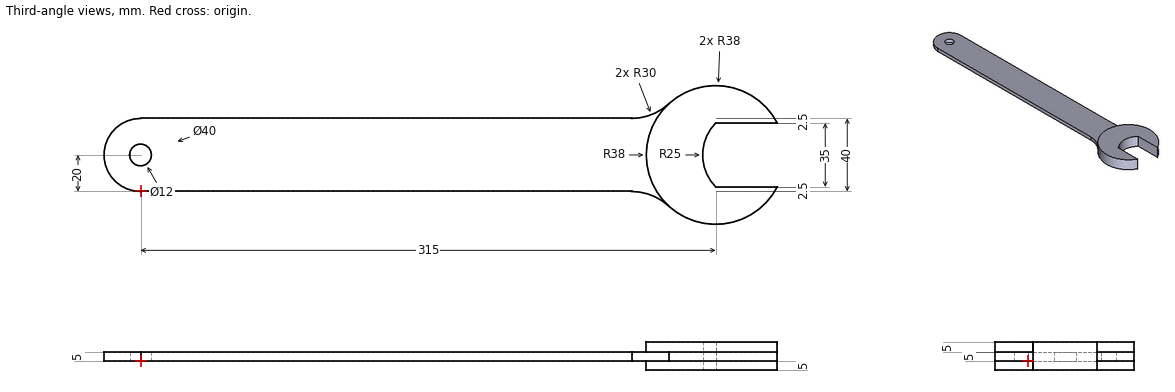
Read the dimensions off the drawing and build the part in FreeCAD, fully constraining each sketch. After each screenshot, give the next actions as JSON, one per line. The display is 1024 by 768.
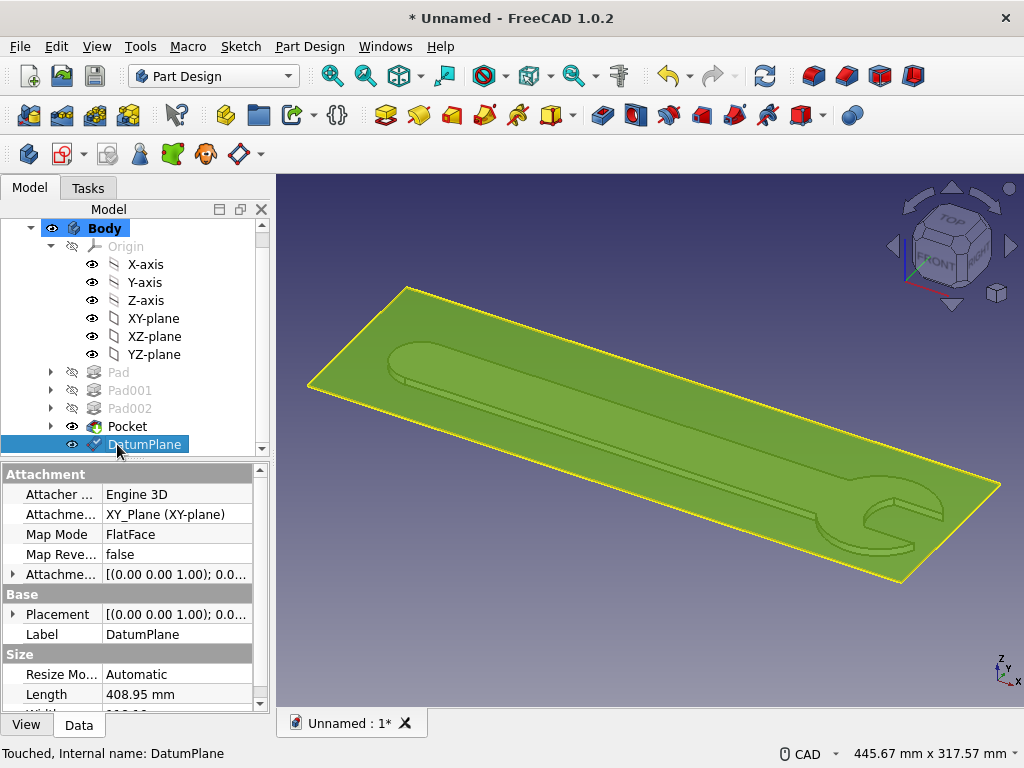
{"action": "left_click", "coordinate": [62, 154]}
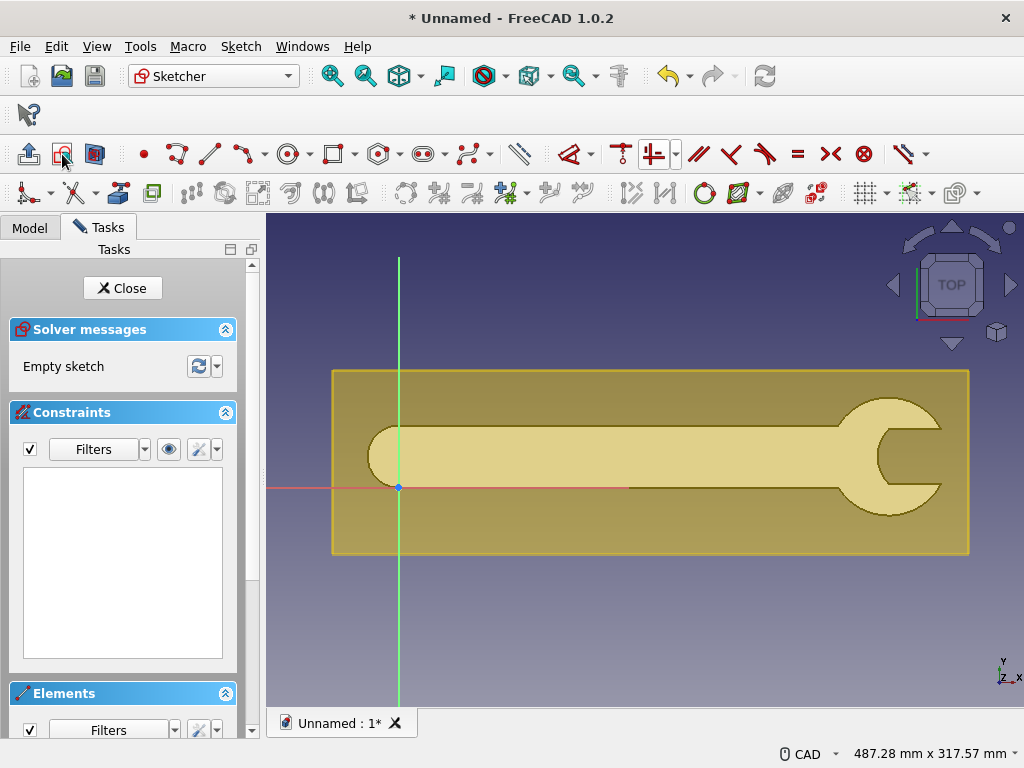
{"action": "scroll", "coordinate": [576, 460], "scroll_direction": "down", "scroll_amount": 5}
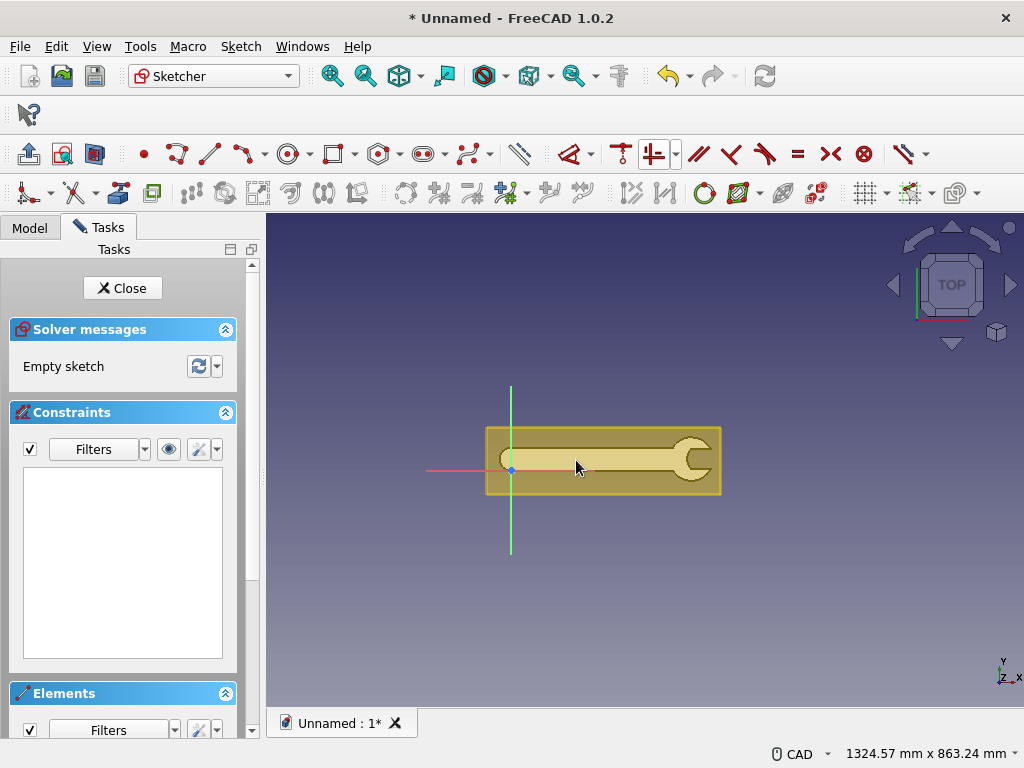
{"action": "scroll", "coordinate": [704, 459], "scroll_direction": "up", "scroll_amount": 11}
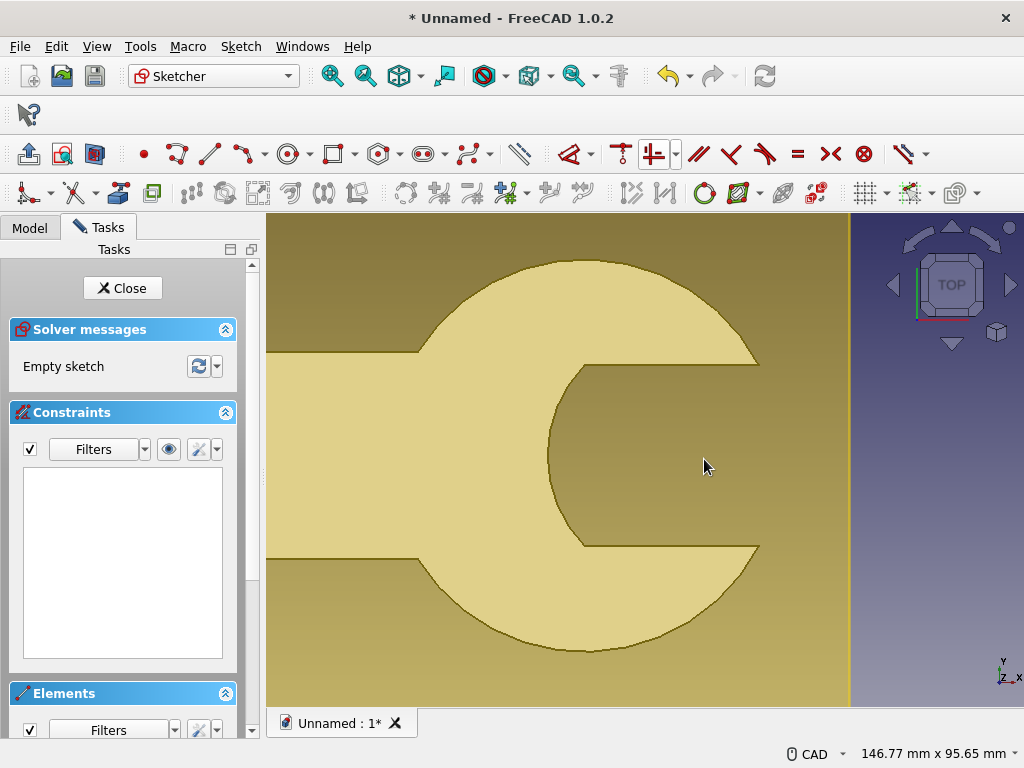
{"action": "left_click", "coordinate": [210, 154]}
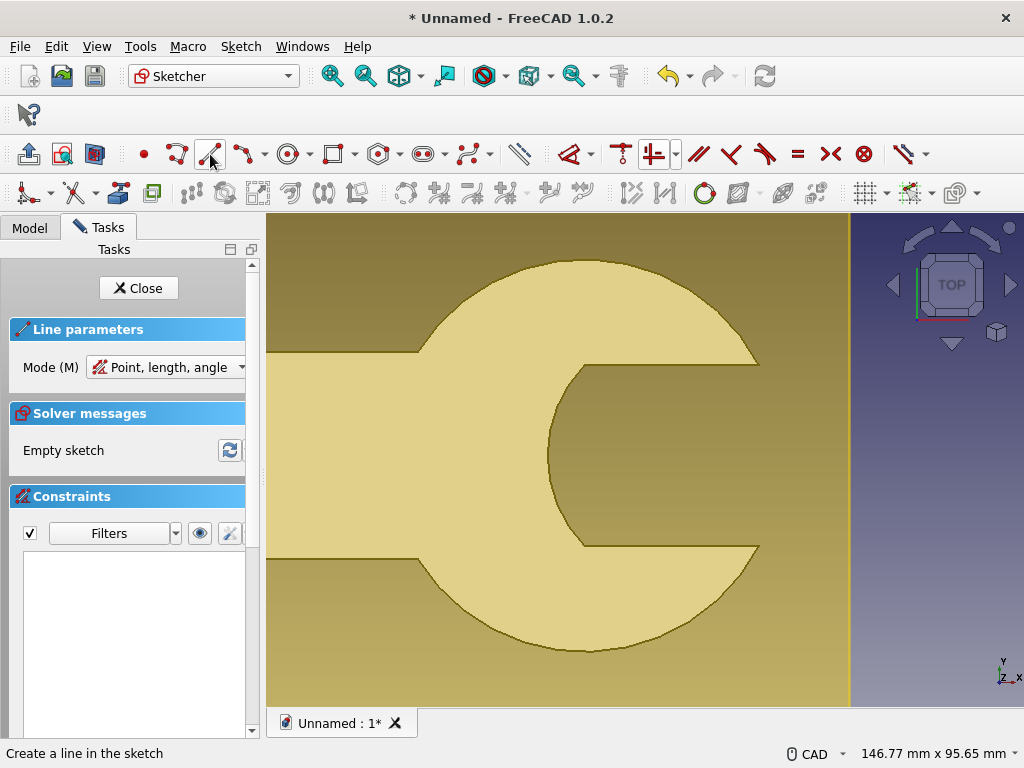
{"action": "left_click", "coordinate": [585, 365]}
{"action": "left_click", "coordinate": [759, 365]}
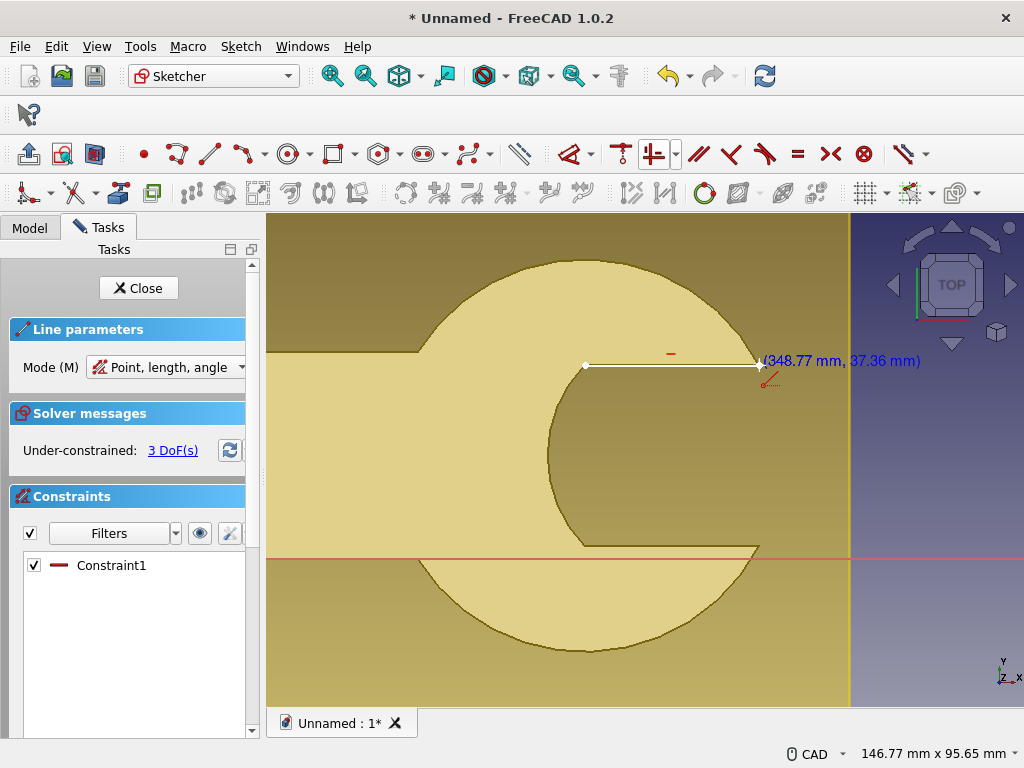
{"action": "scroll", "coordinate": [759, 546], "scroll_direction": "up", "scroll_amount": 2}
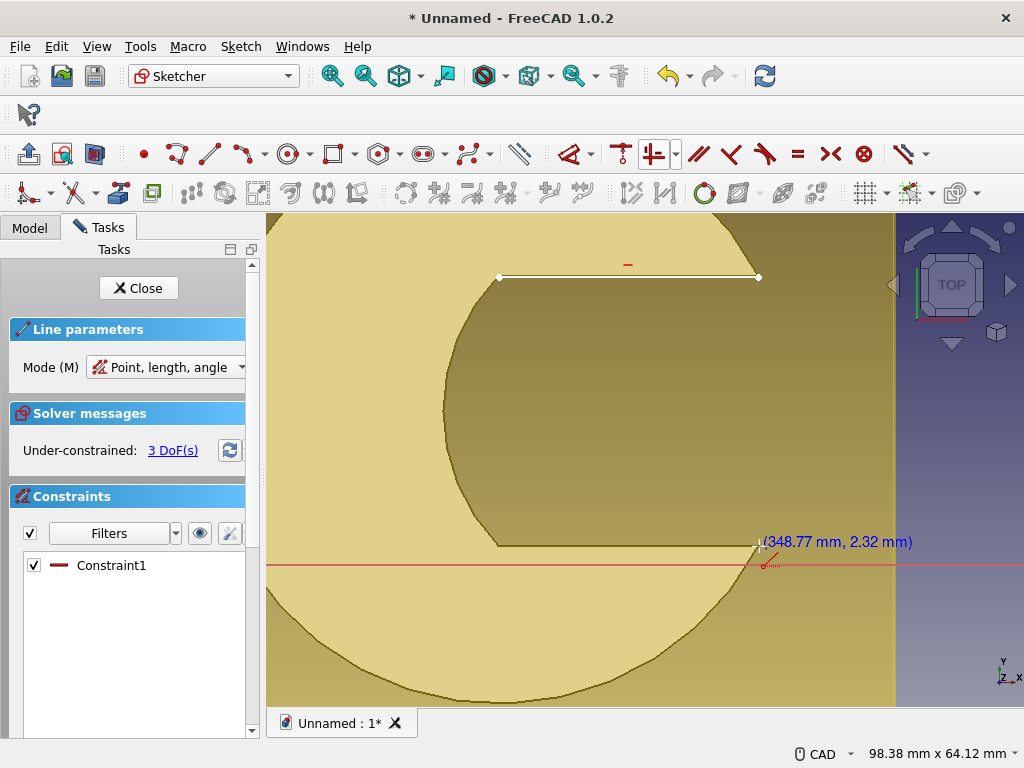
{"action": "left_click", "coordinate": [758, 546]}
{"action": "left_click", "coordinate": [498, 546]}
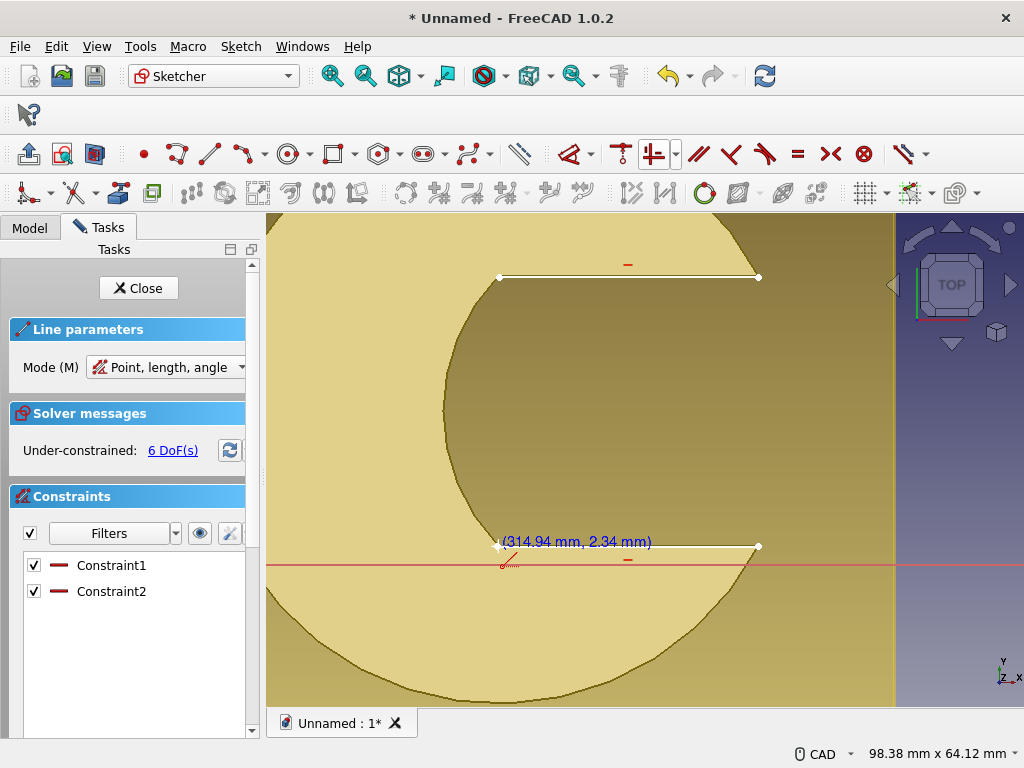
{"action": "left_click", "coordinate": [242, 154]}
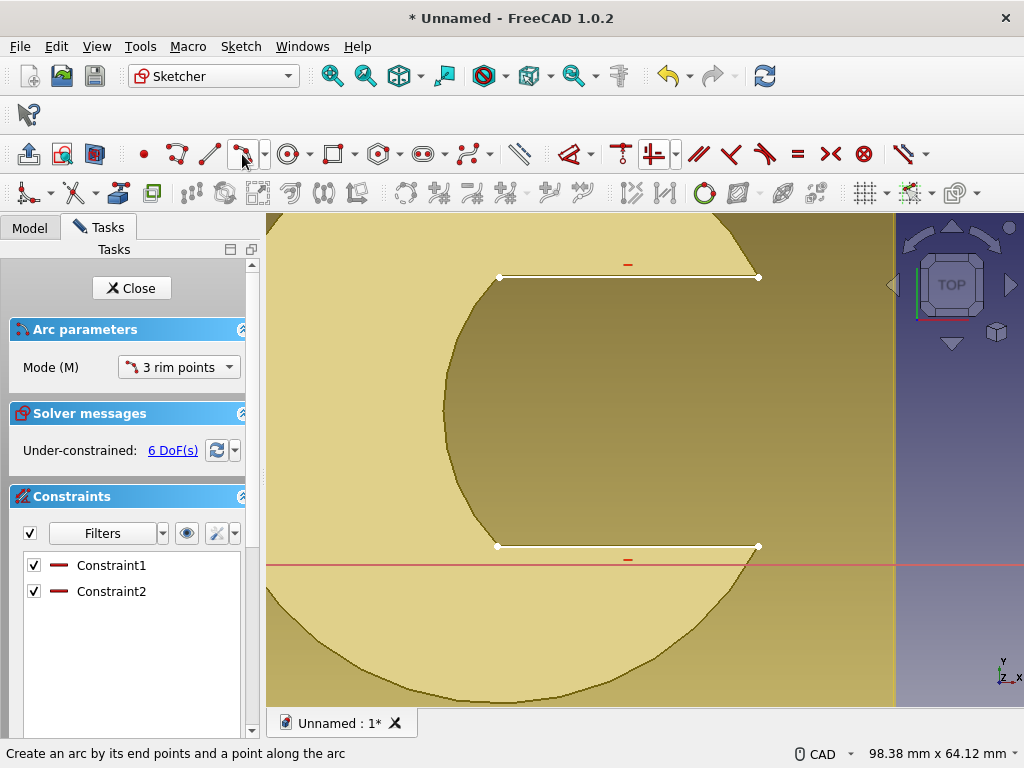
{"action": "left_click", "coordinate": [759, 277]}
{"action": "left_click", "coordinate": [758, 547]}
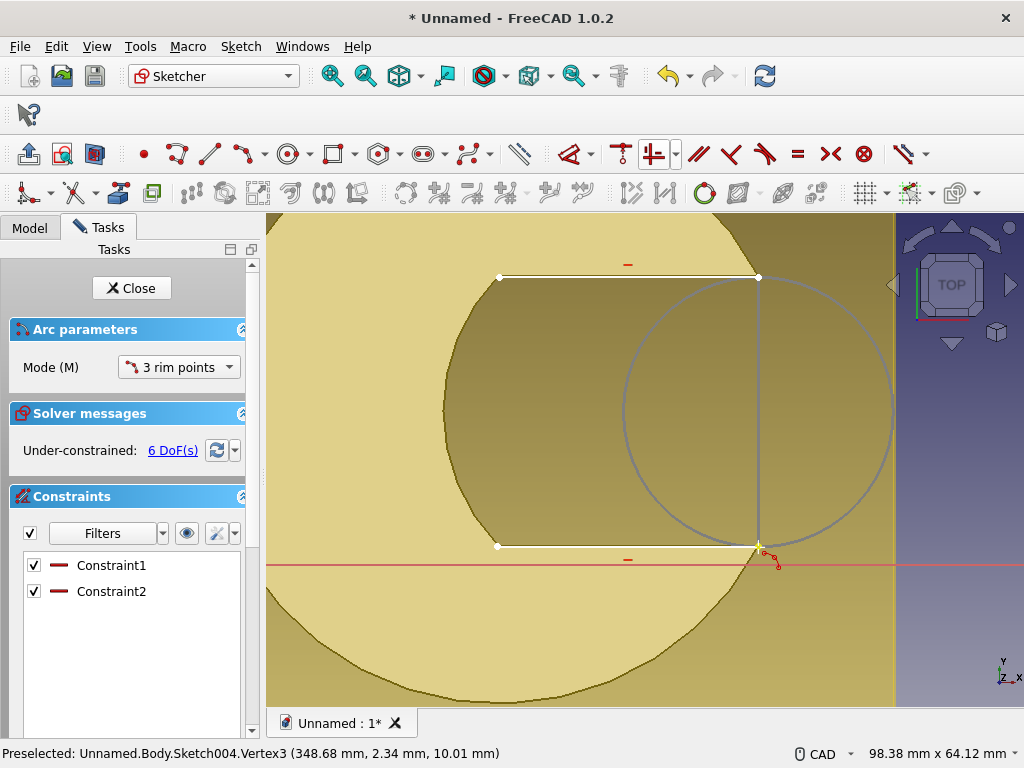
{"action": "scroll", "coordinate": [769, 560], "scroll_direction": "down", "scroll_amount": 2}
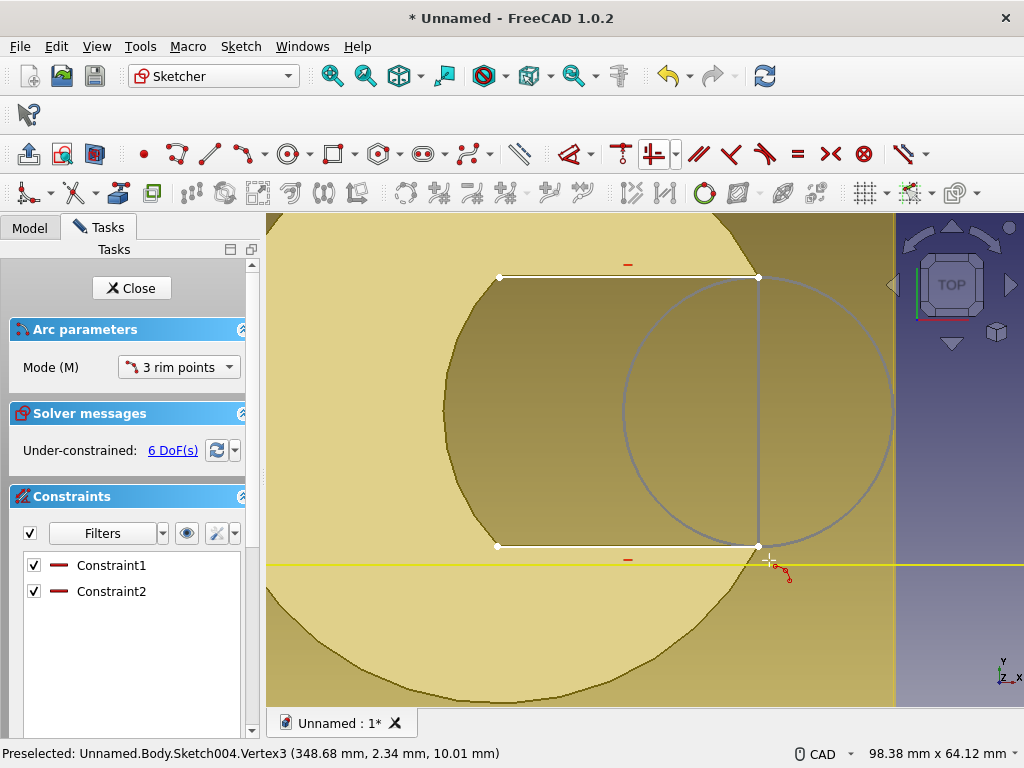
{"action": "left_click", "coordinate": [392, 460]}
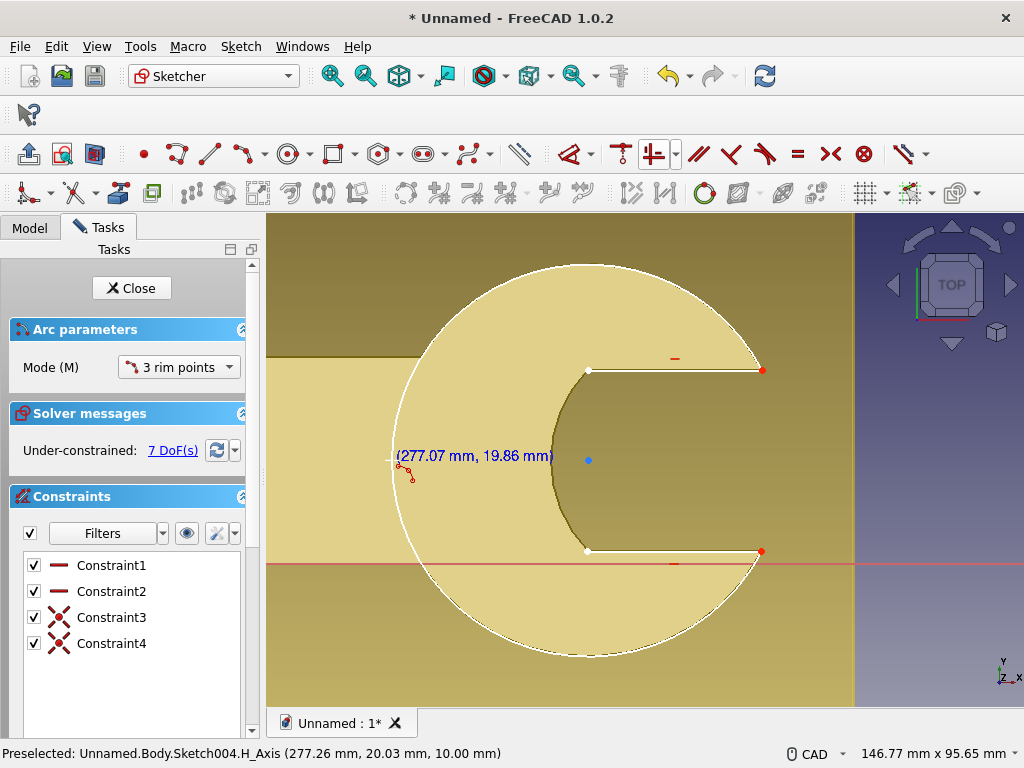
{"action": "scroll", "coordinate": [588, 551], "scroll_direction": "up", "scroll_amount": 2}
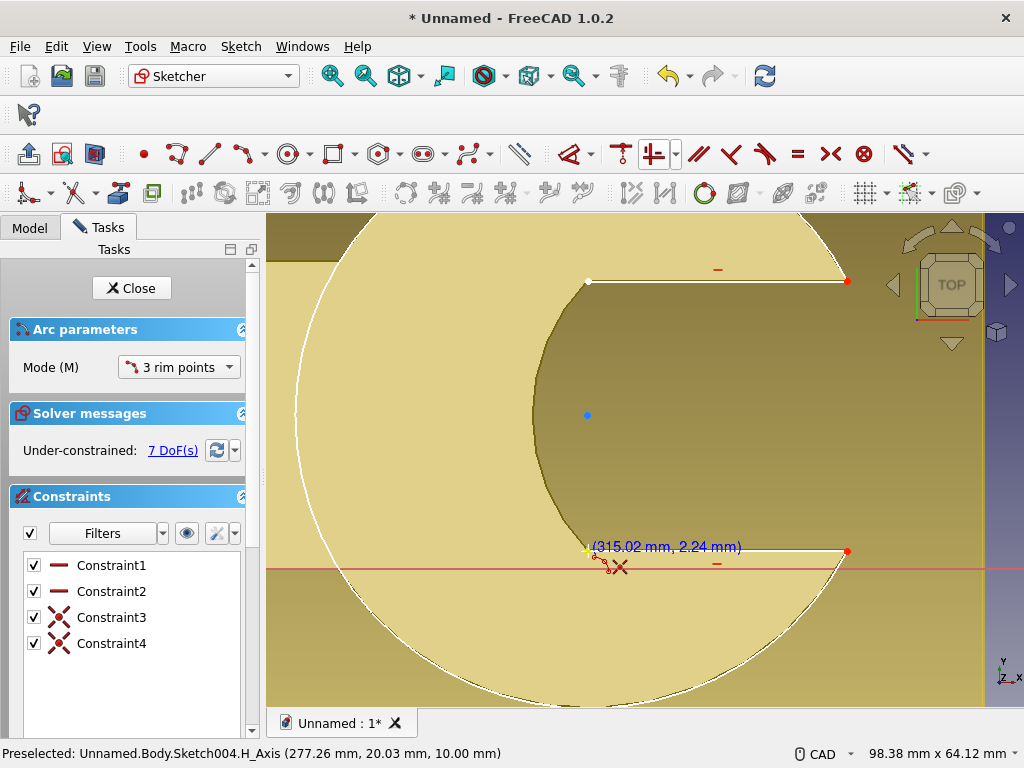
{"action": "left_click", "coordinate": [587, 551]}
{"action": "left_click", "coordinate": [588, 282]}
{"action": "left_click", "coordinate": [533, 415]}
{"action": "key", "text": "Escape"}